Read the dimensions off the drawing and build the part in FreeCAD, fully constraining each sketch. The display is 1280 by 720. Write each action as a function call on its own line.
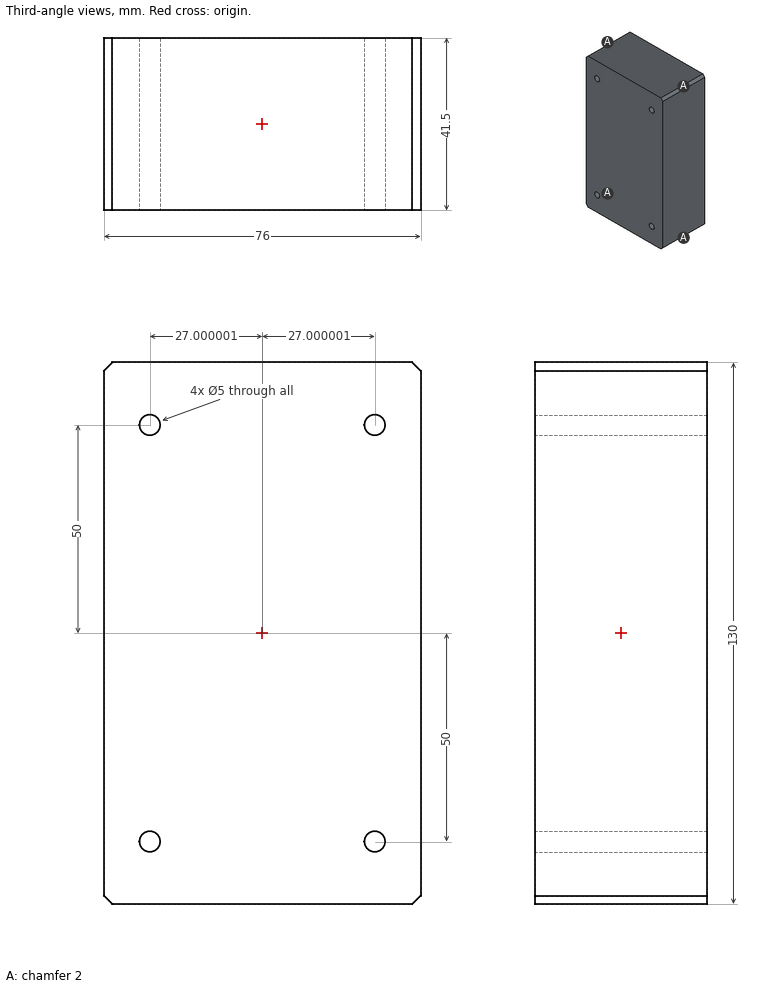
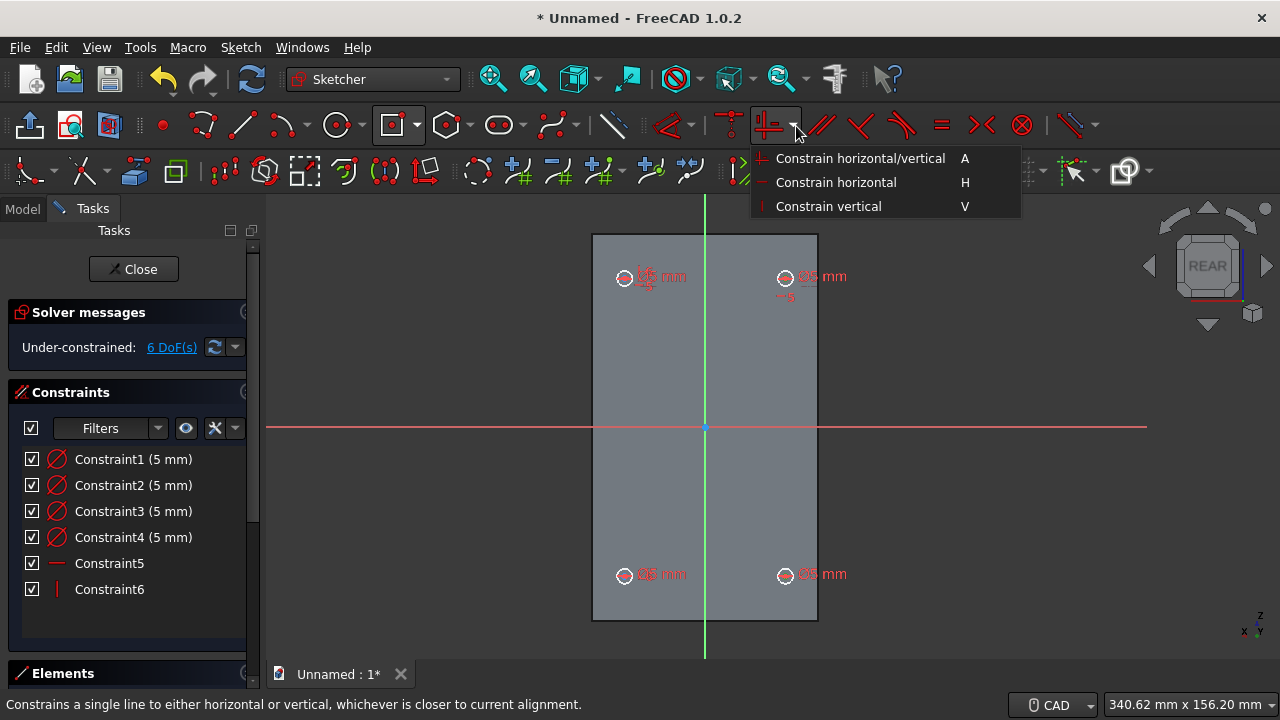
click(886, 206)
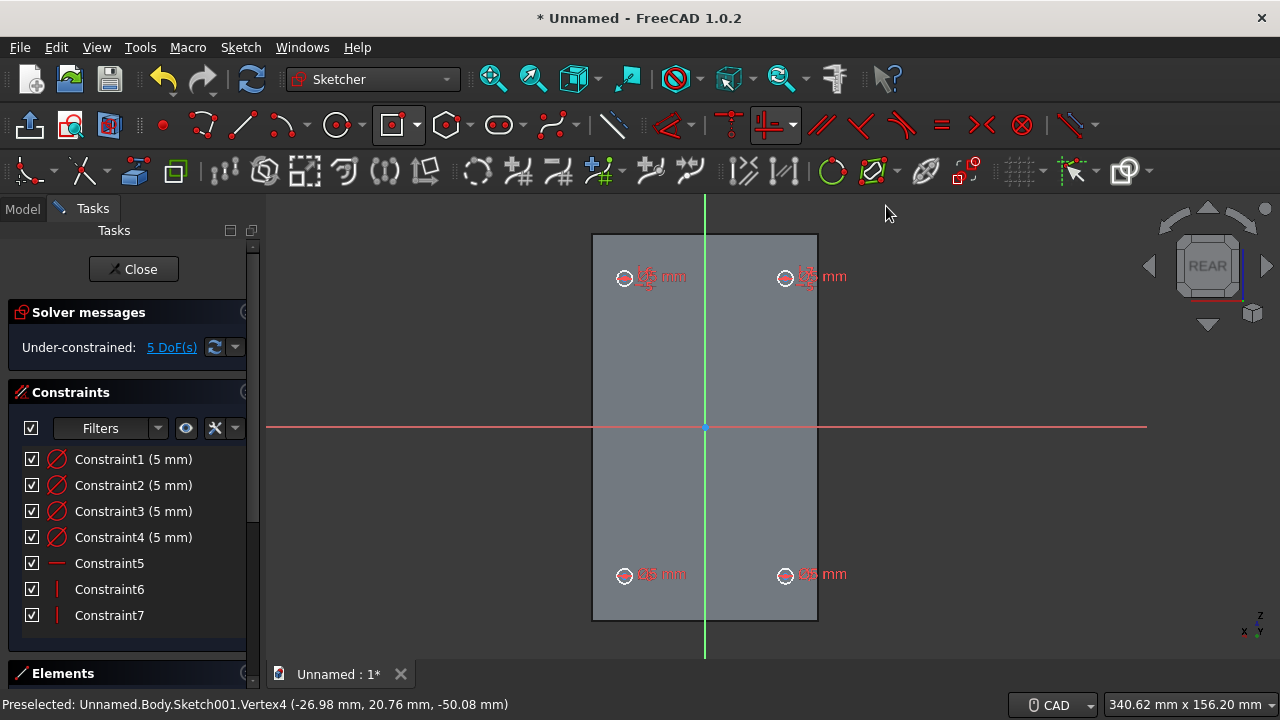
click(625, 576)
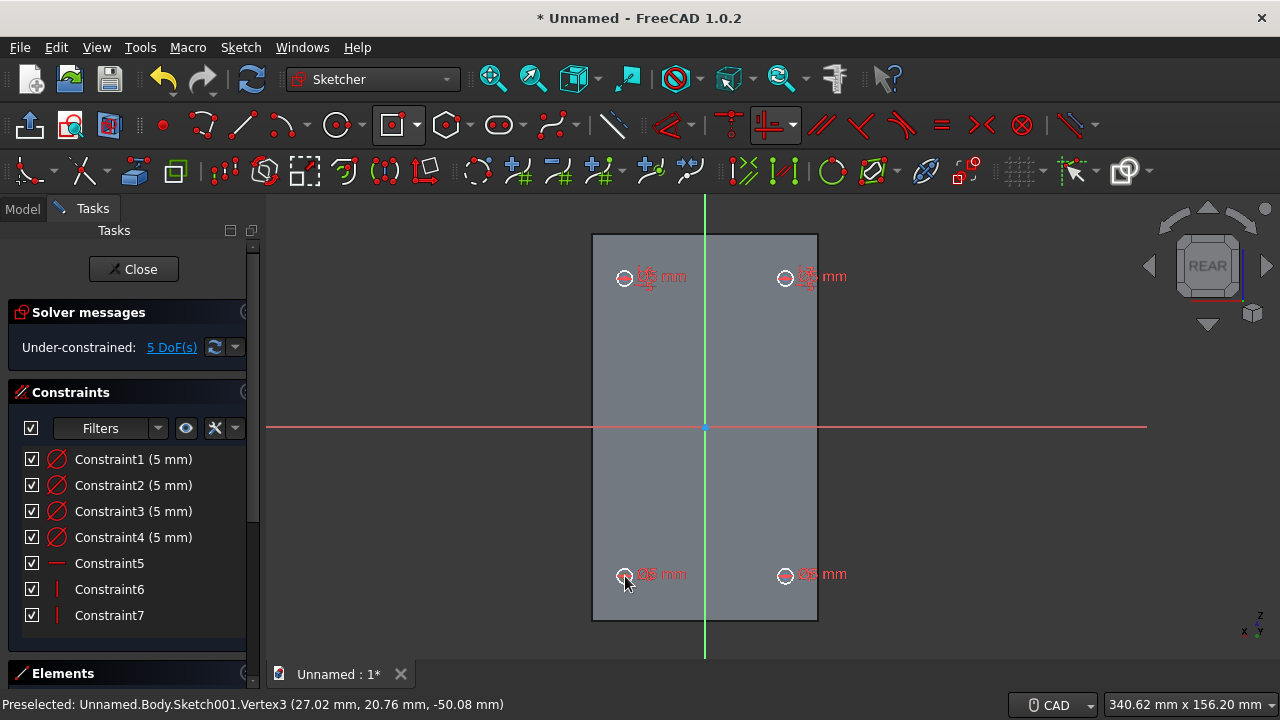
click(786, 576)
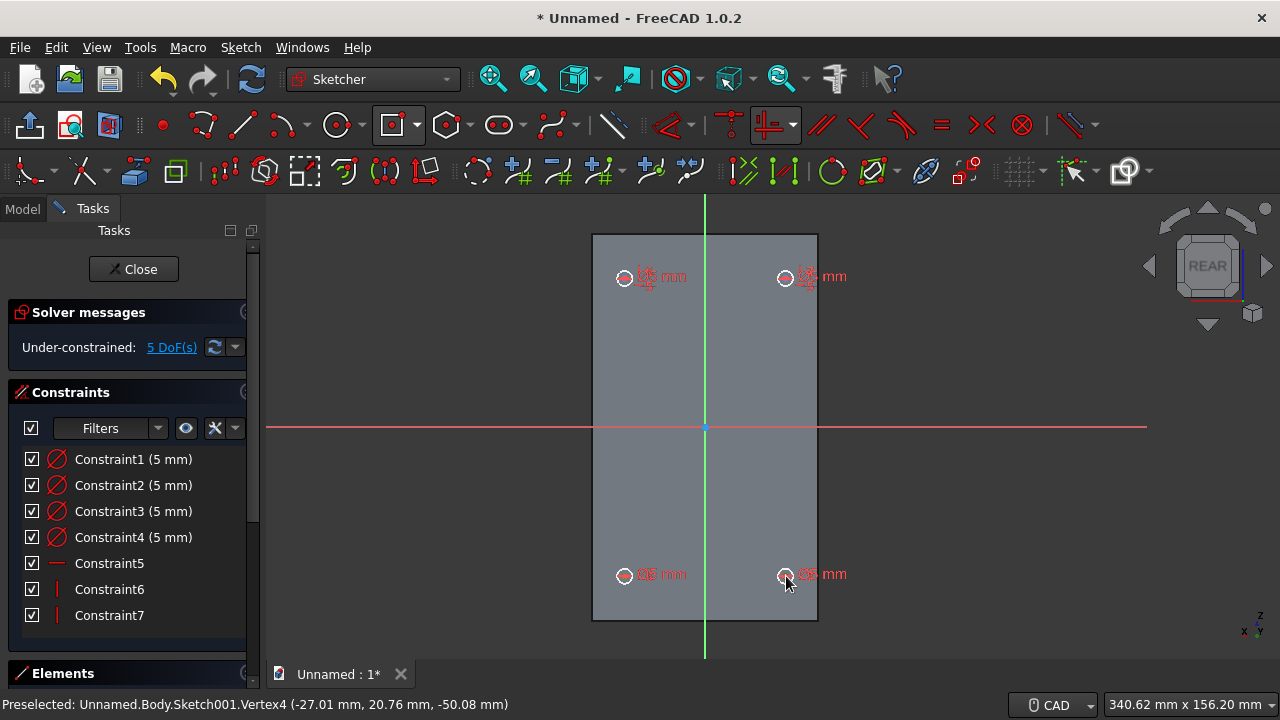
click(796, 126)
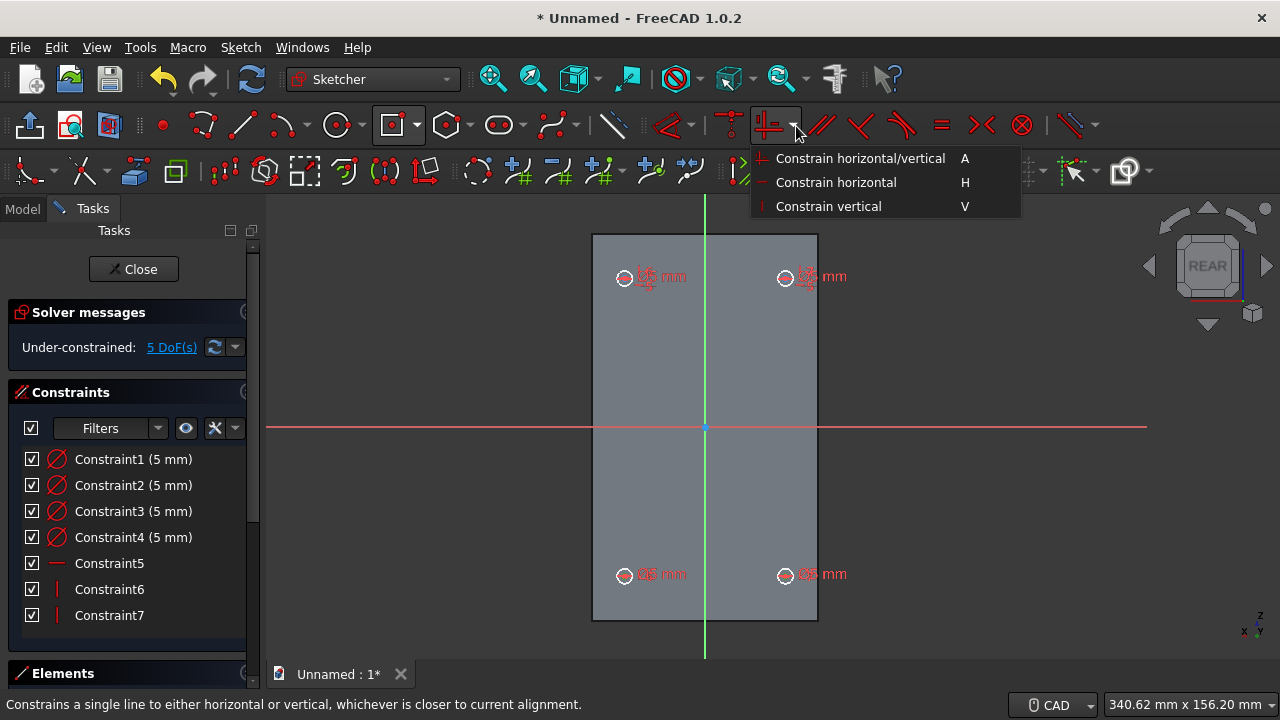
click(886, 182)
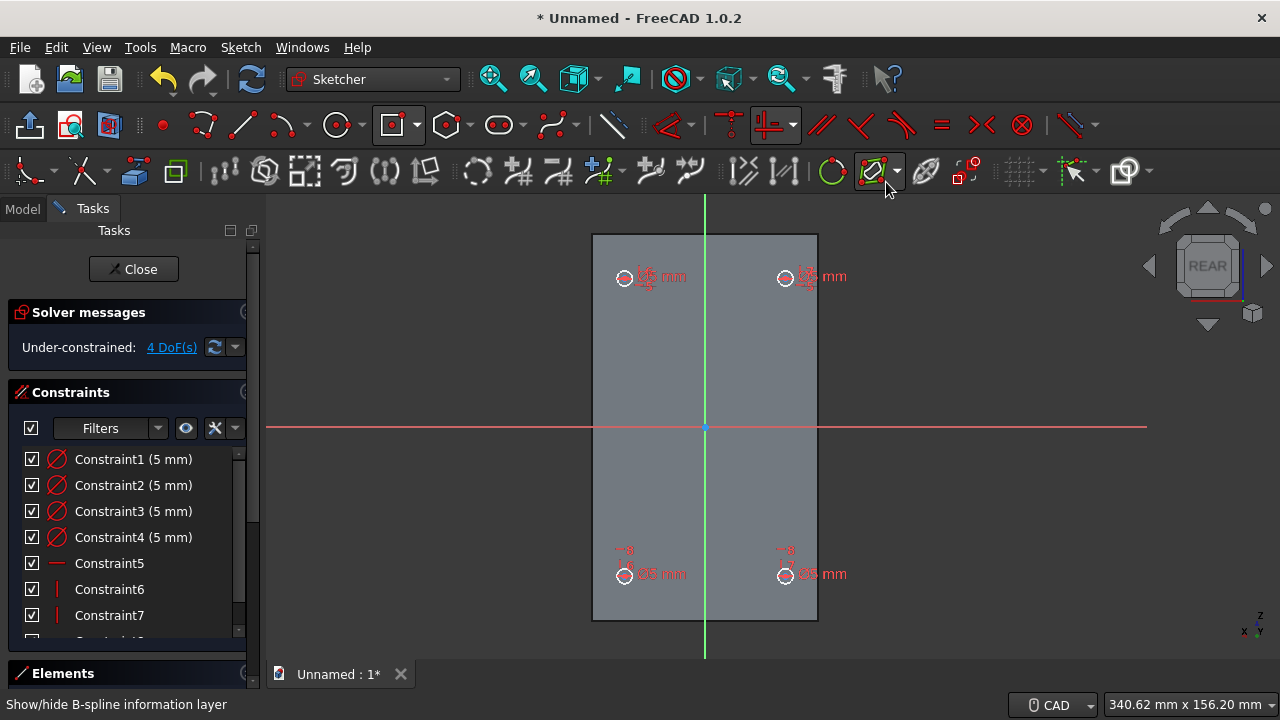
click(668, 126)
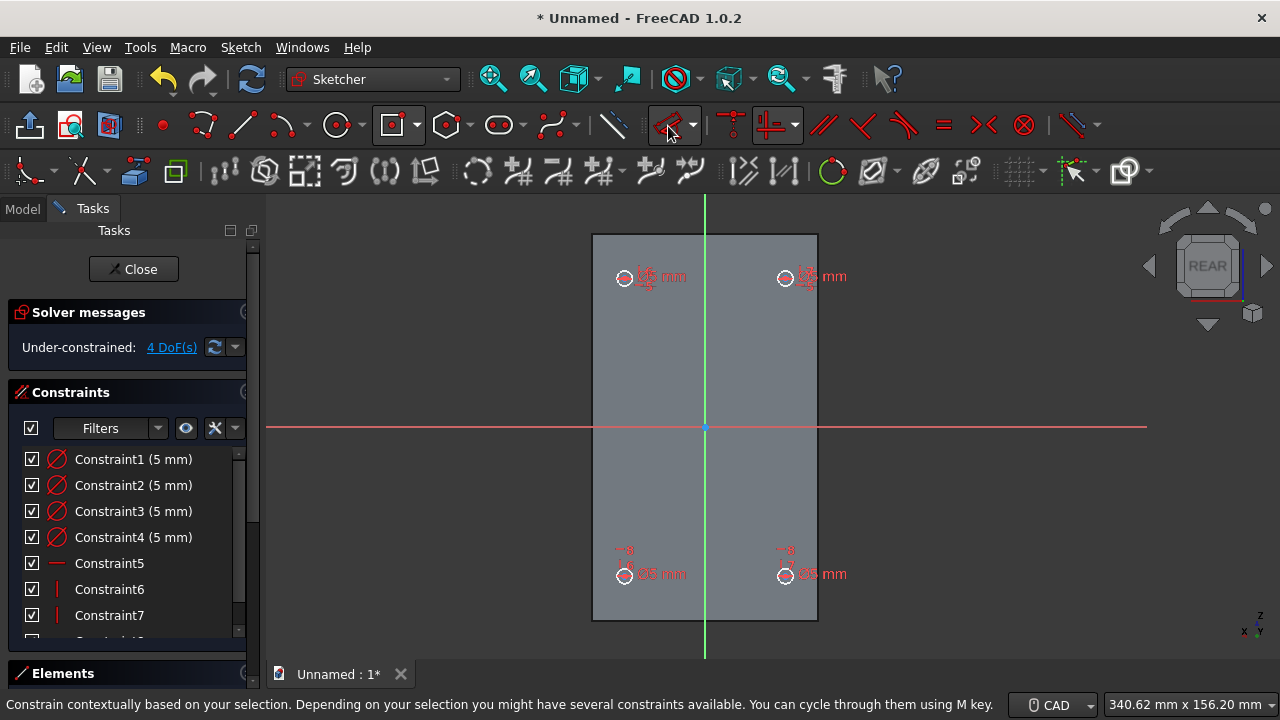
click(786, 279)
click(820, 353)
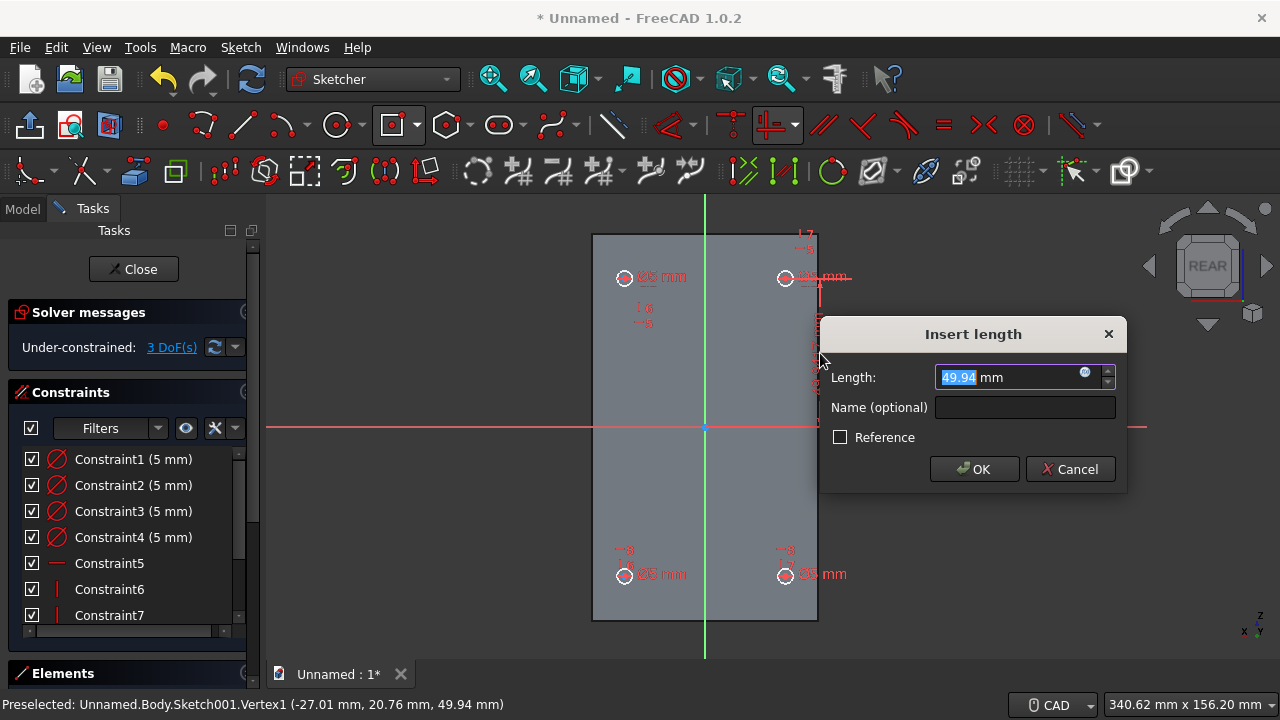
text(50)
key(Return)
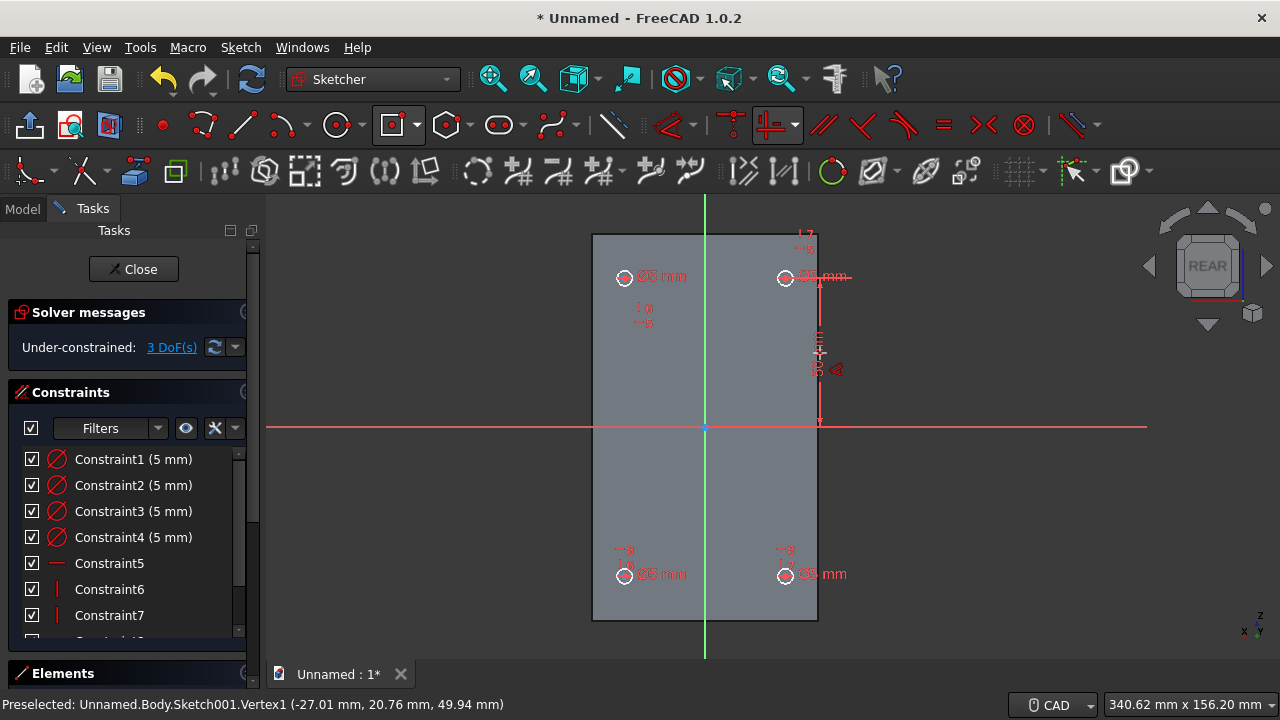
click(625, 576)
click(591, 502)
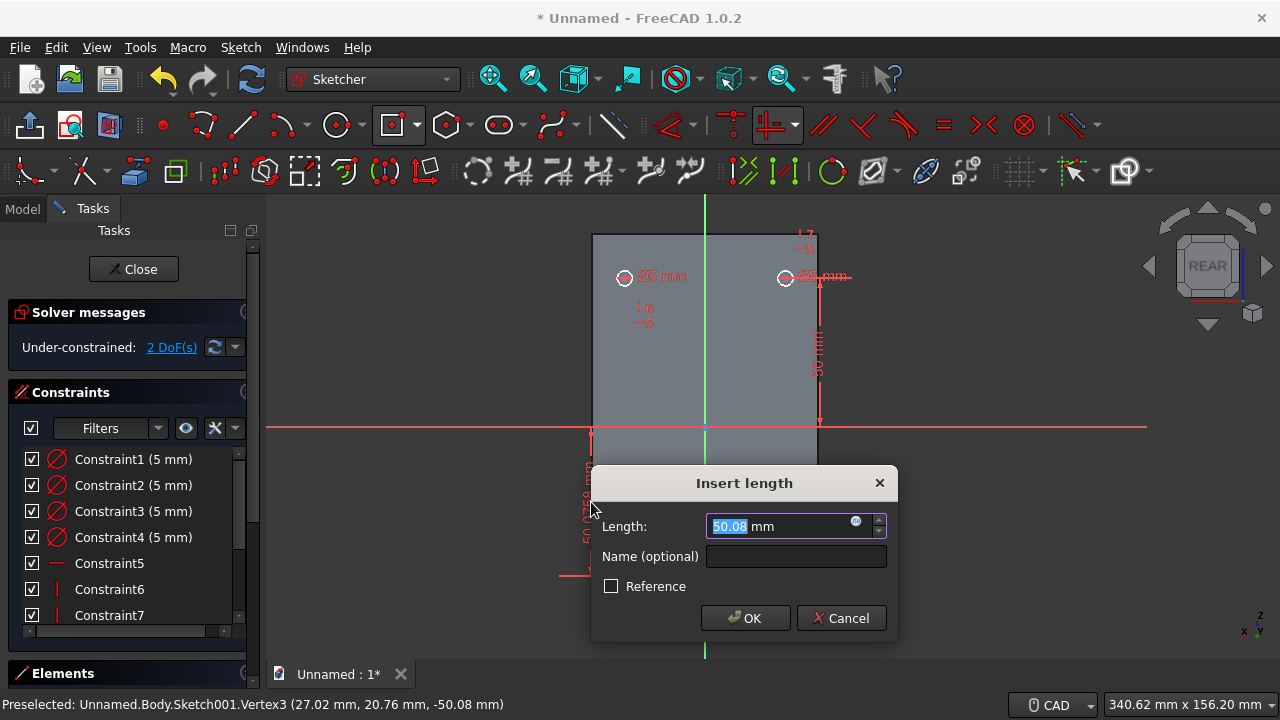
text(50)
key(Return)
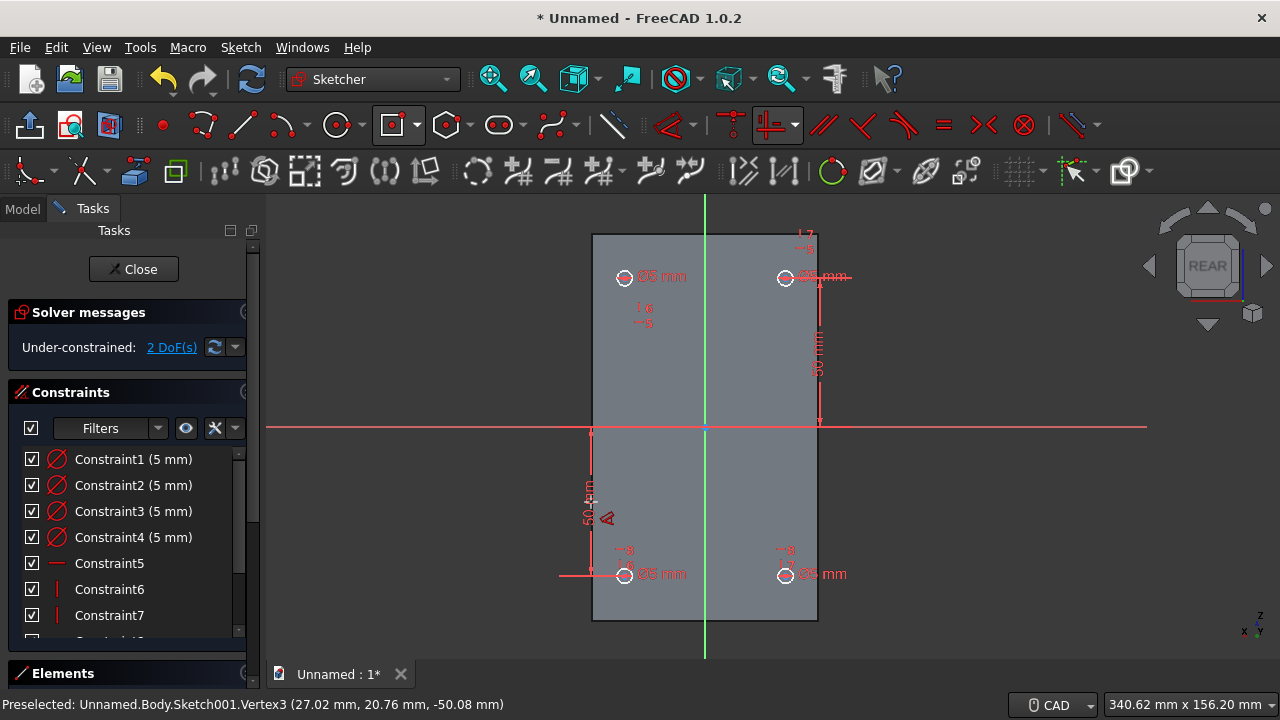
click(786, 278)
click(745, 244)